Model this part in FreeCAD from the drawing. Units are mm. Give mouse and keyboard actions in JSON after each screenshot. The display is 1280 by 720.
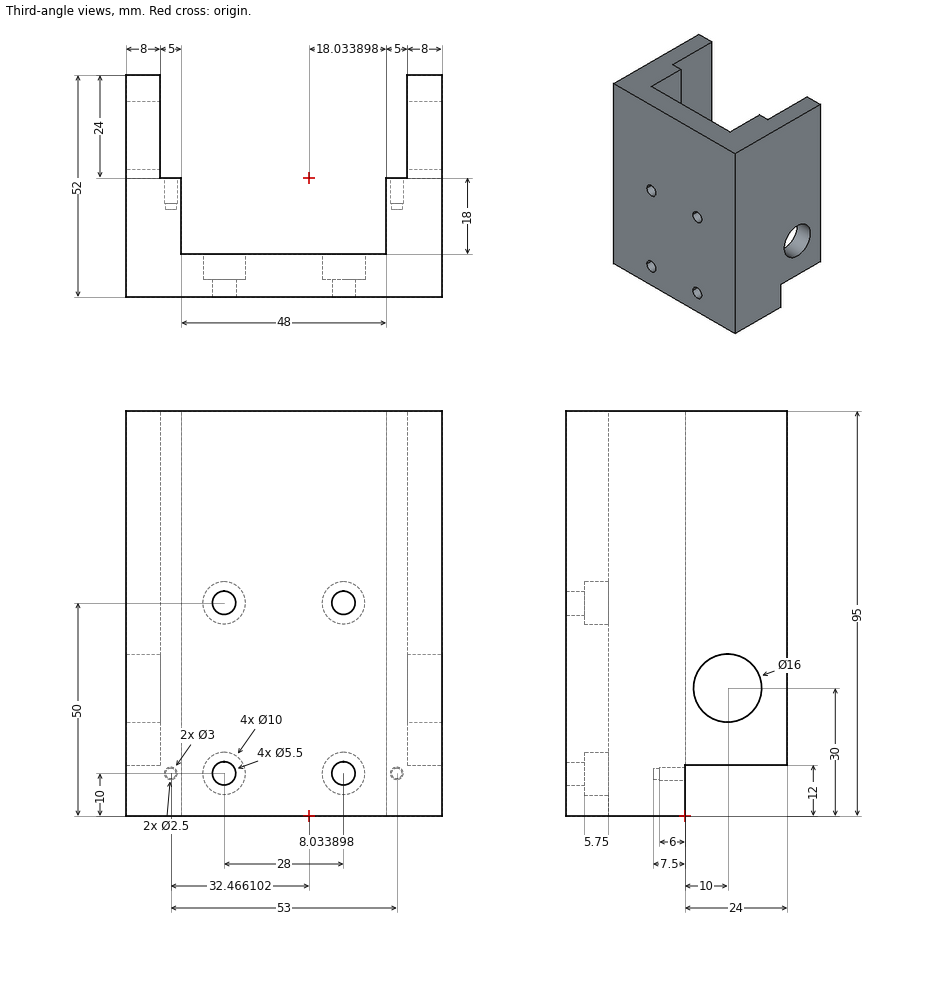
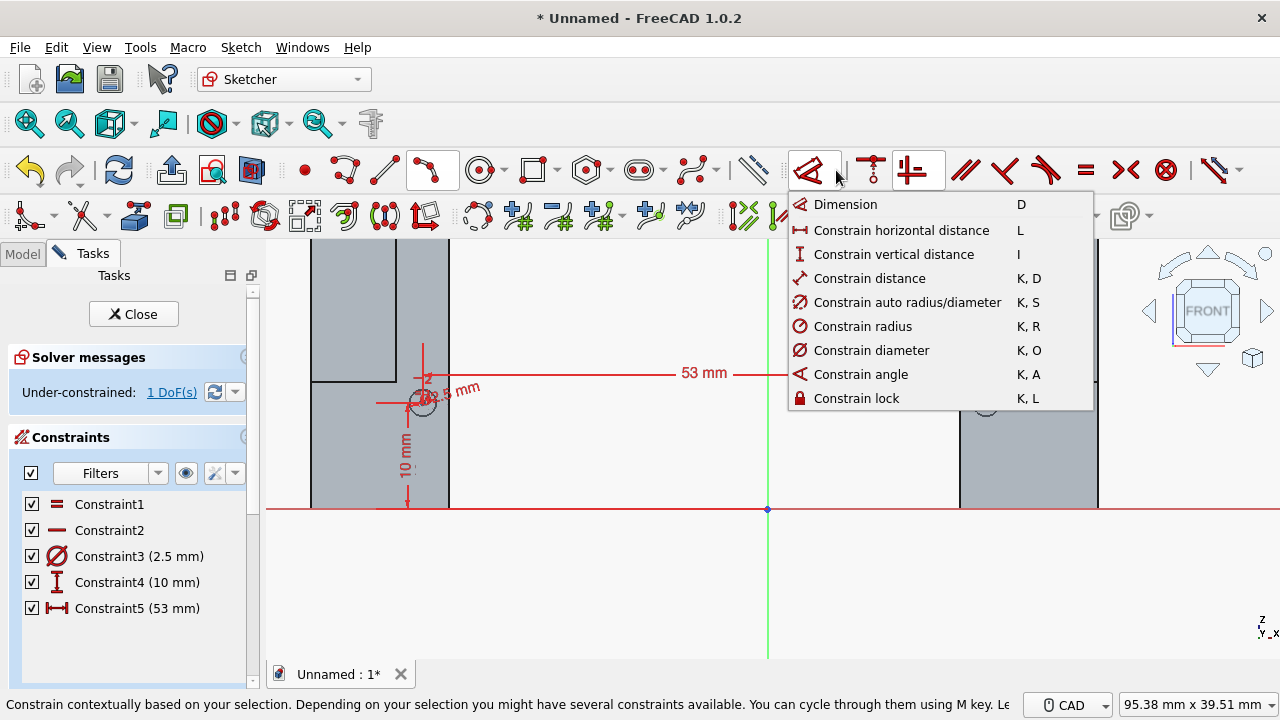
{"action": "left_click", "coordinate": [941, 230]}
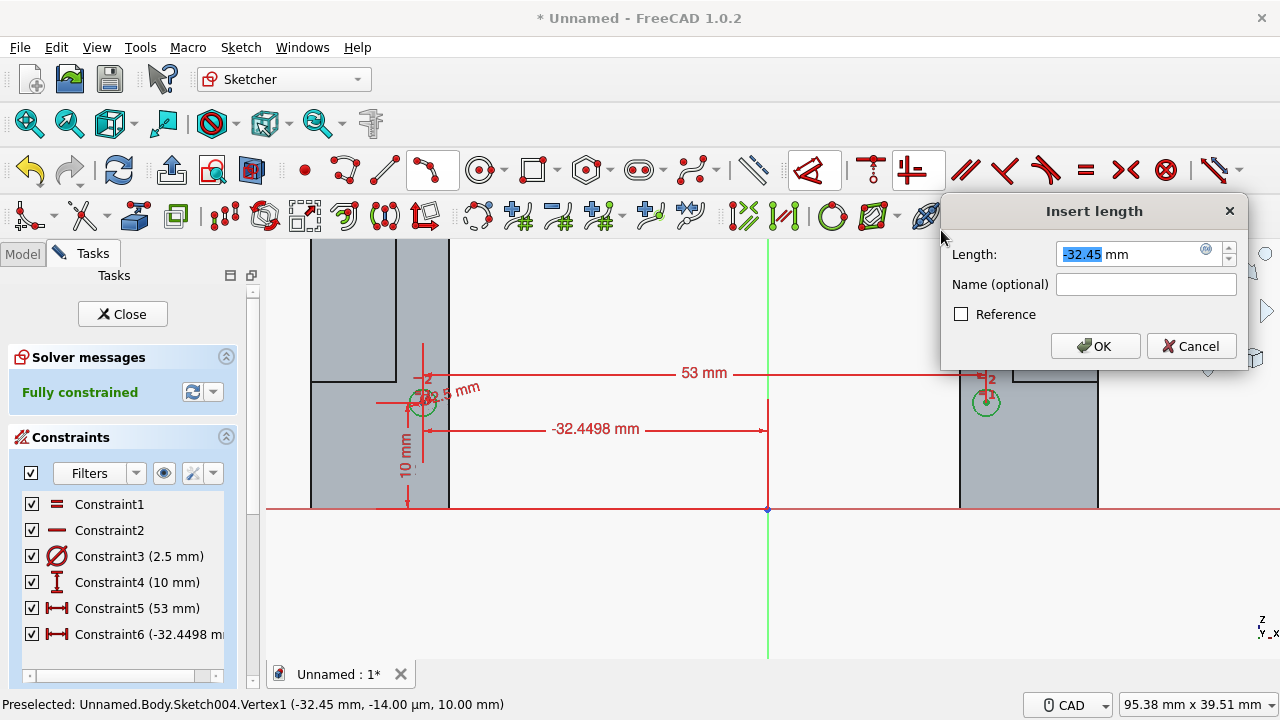
{"action": "type", "text": "-32.466102"}
{"action": "key", "text": "Return"}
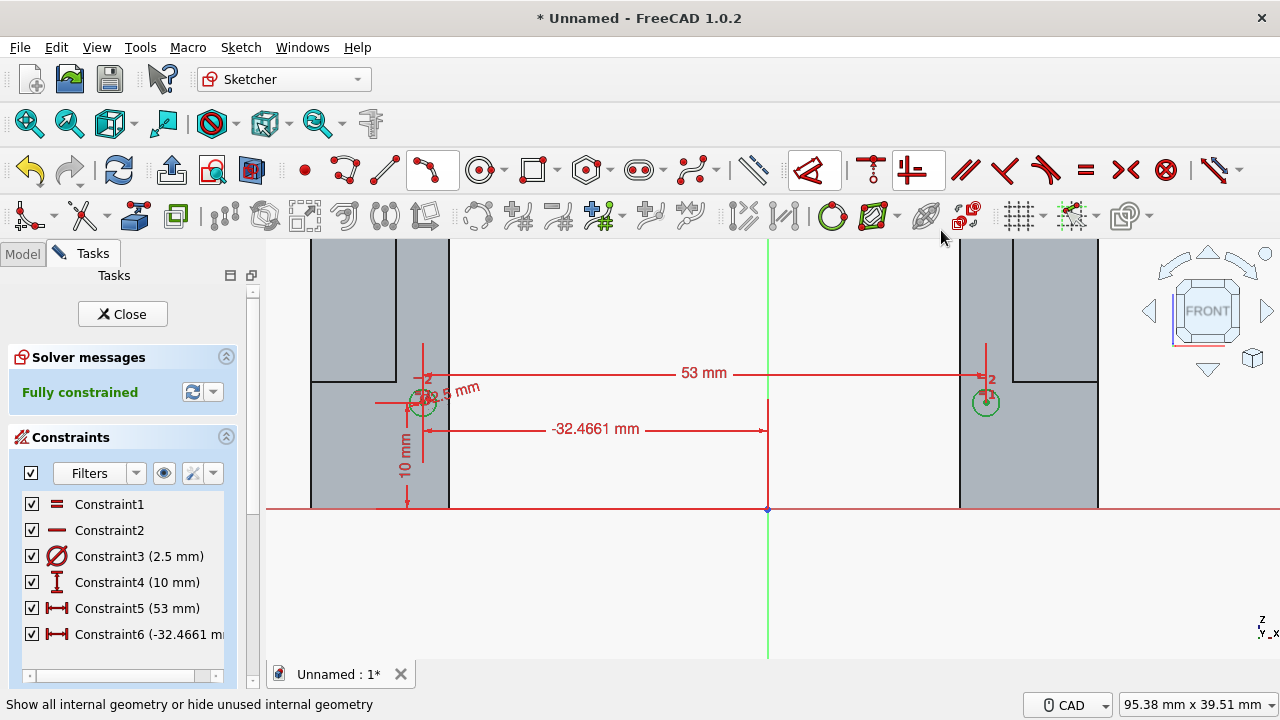
{"action": "left_click", "coordinate": [123, 314]}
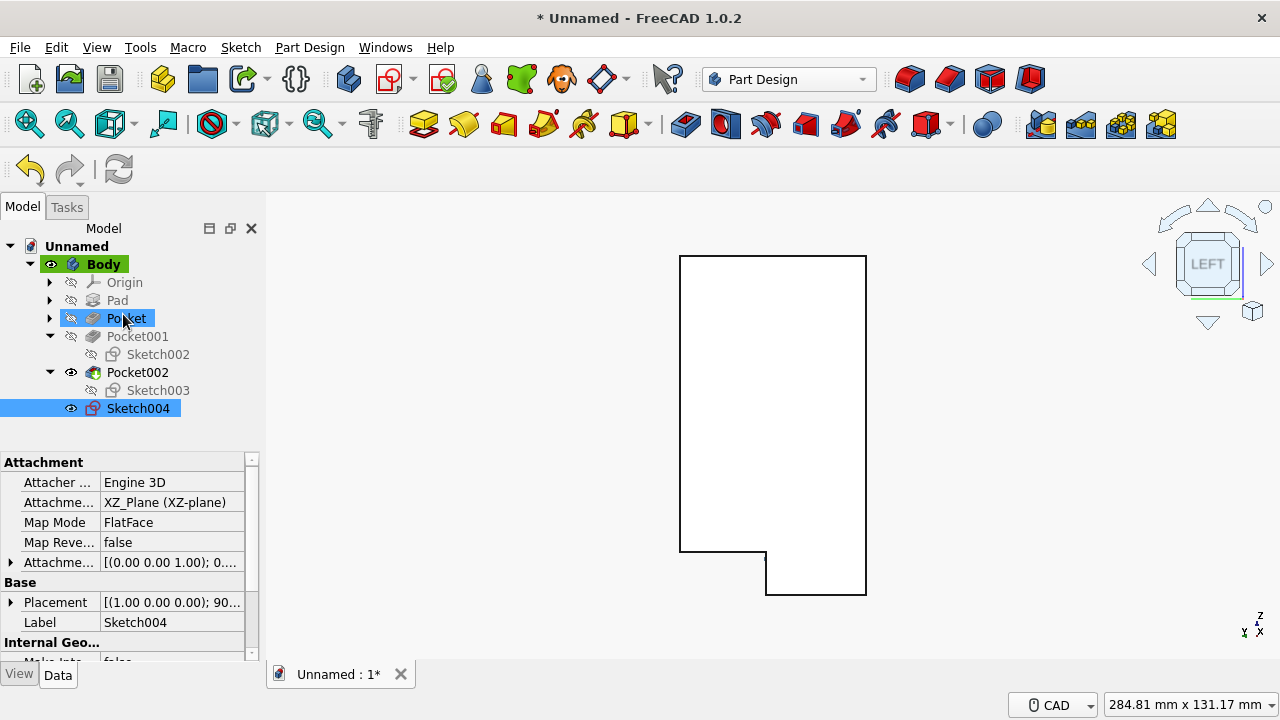
{"action": "left_click", "coordinate": [686, 124]}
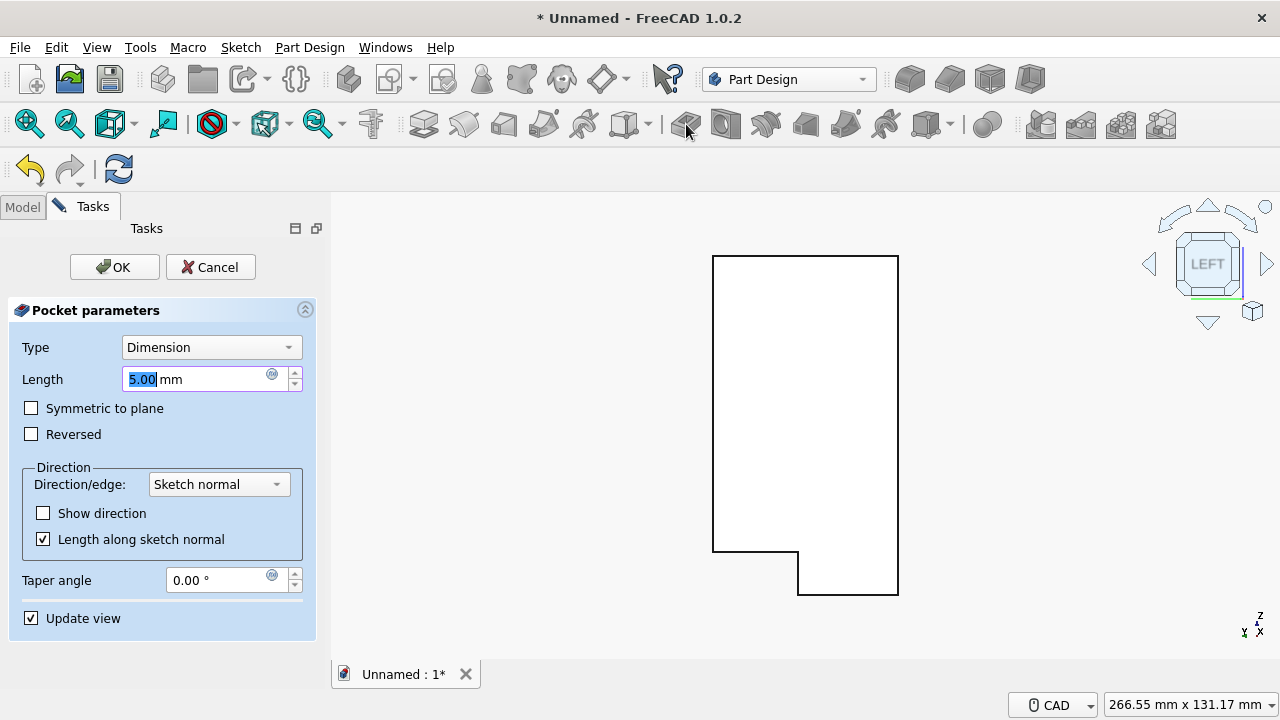
{"action": "type", "text": "7.5"}
{"action": "key", "text": "Tab"}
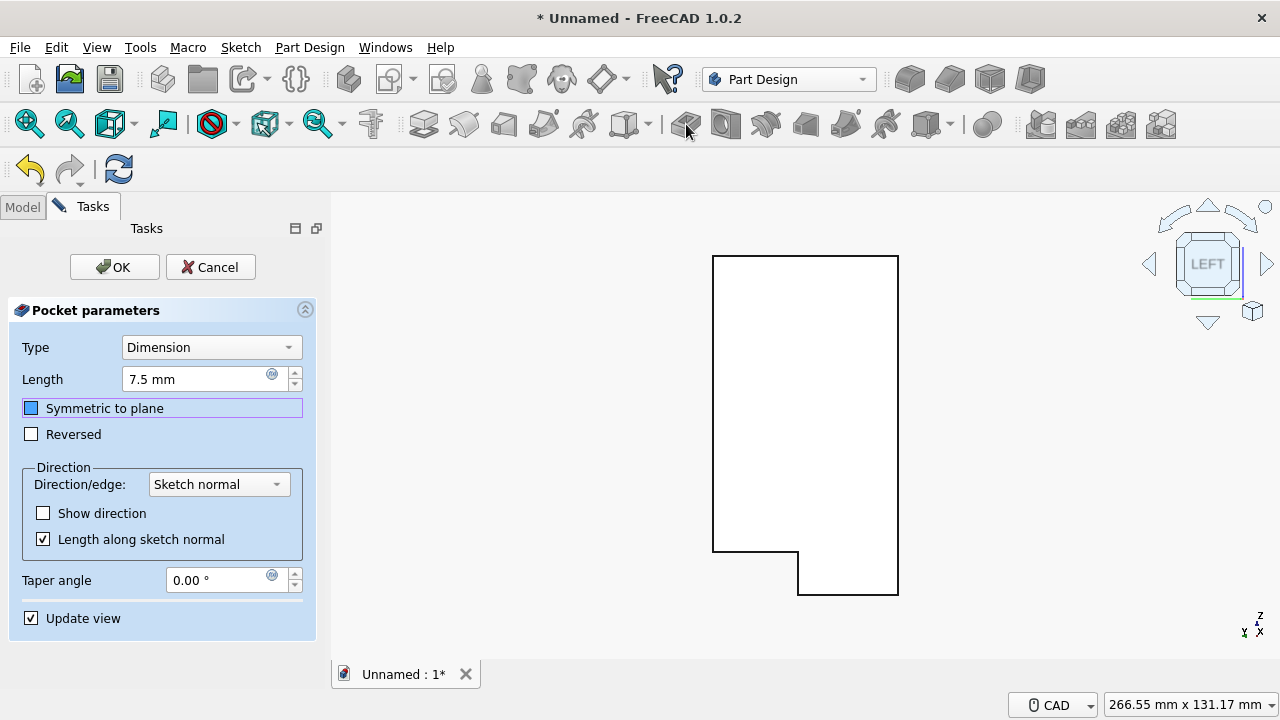
{"action": "left_click", "coordinate": [30, 434]}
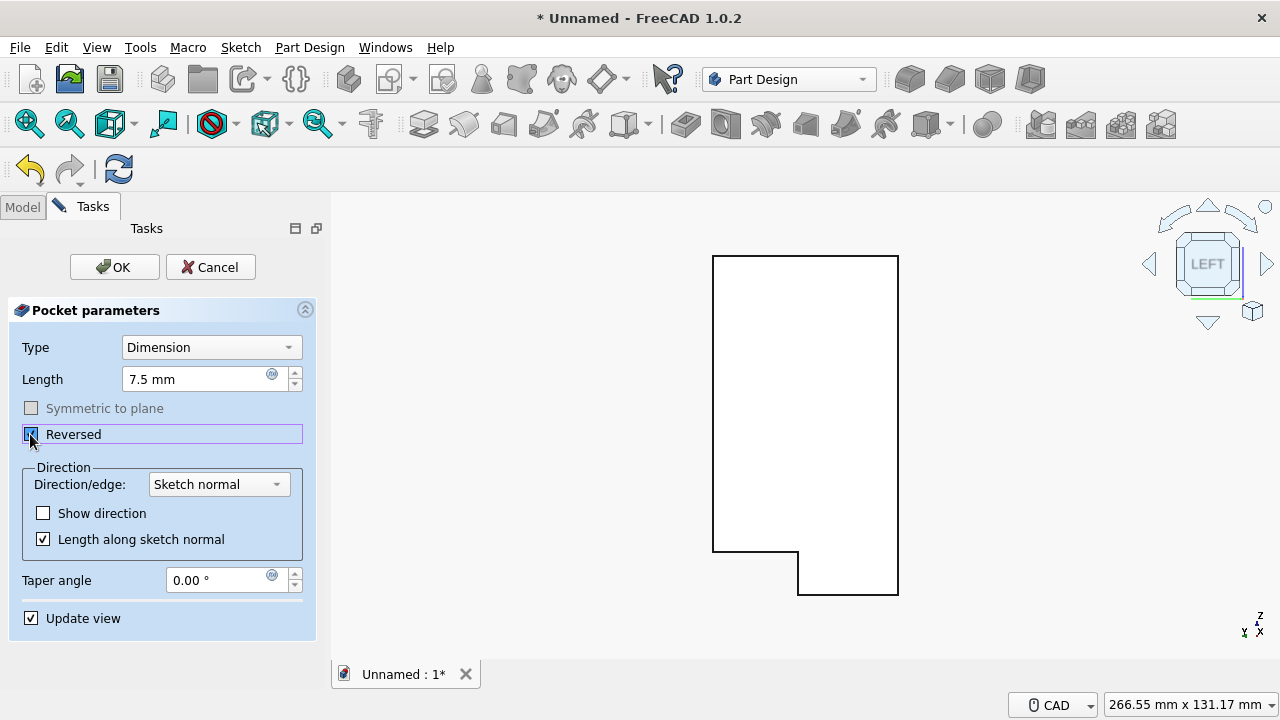
{"action": "left_click", "coordinate": [115, 267]}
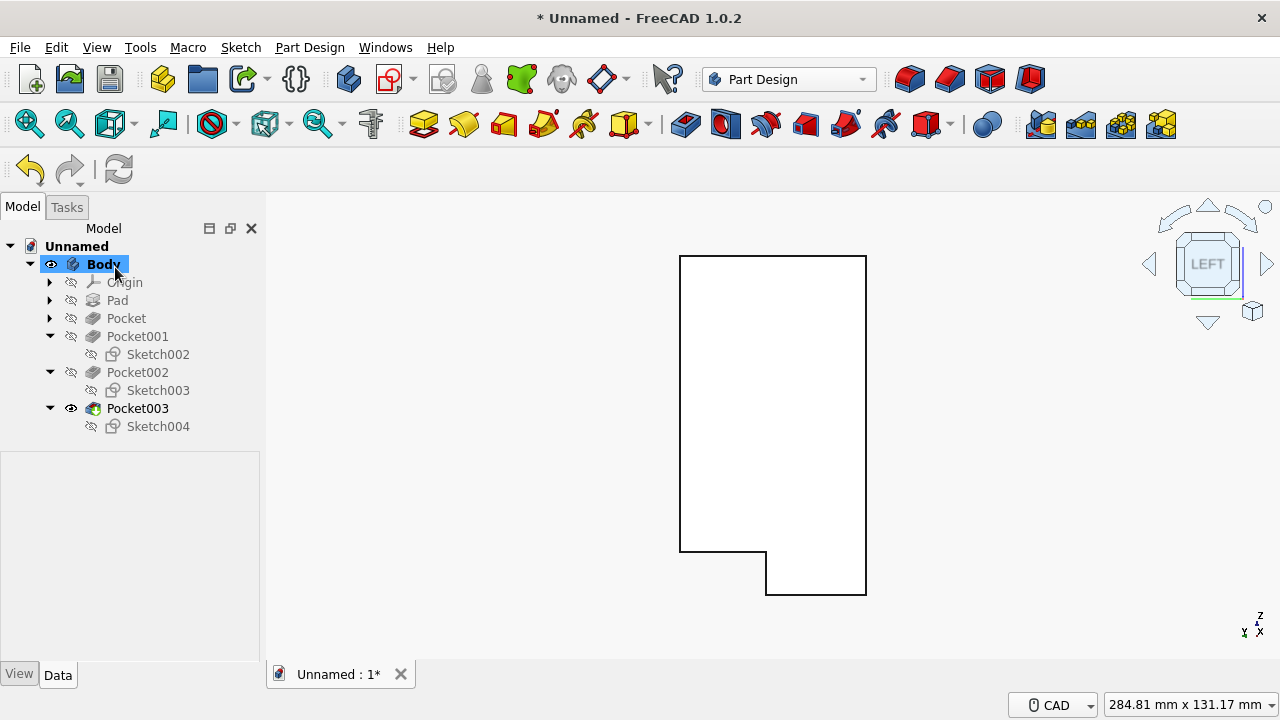
{"action": "key", "text": "4"}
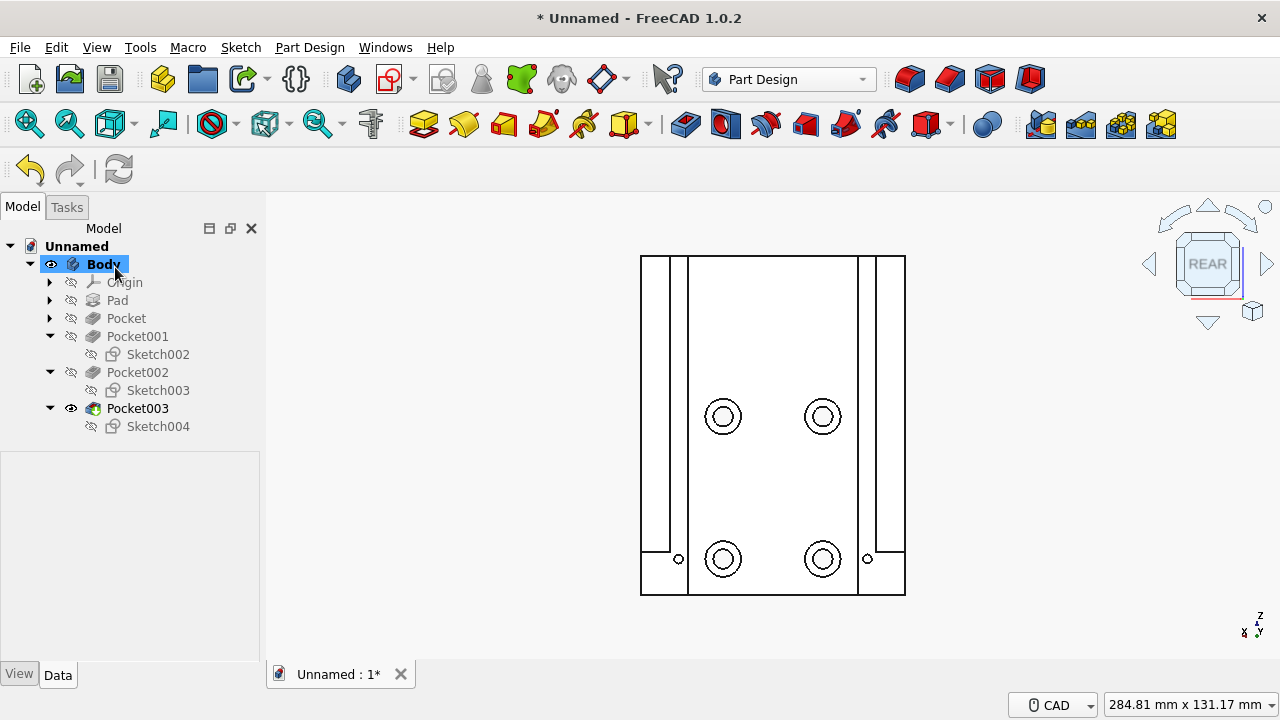
{"action": "left_click", "coordinate": [658, 569]}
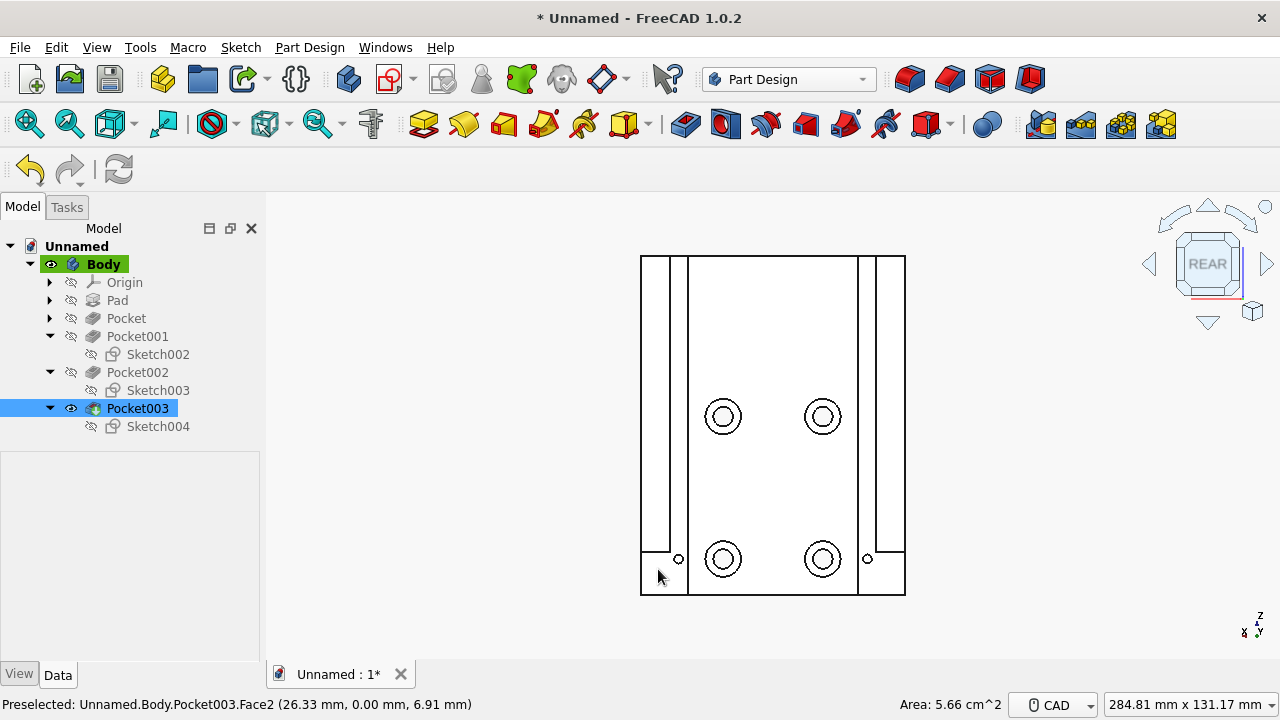
{"action": "left_click", "coordinate": [390, 80]}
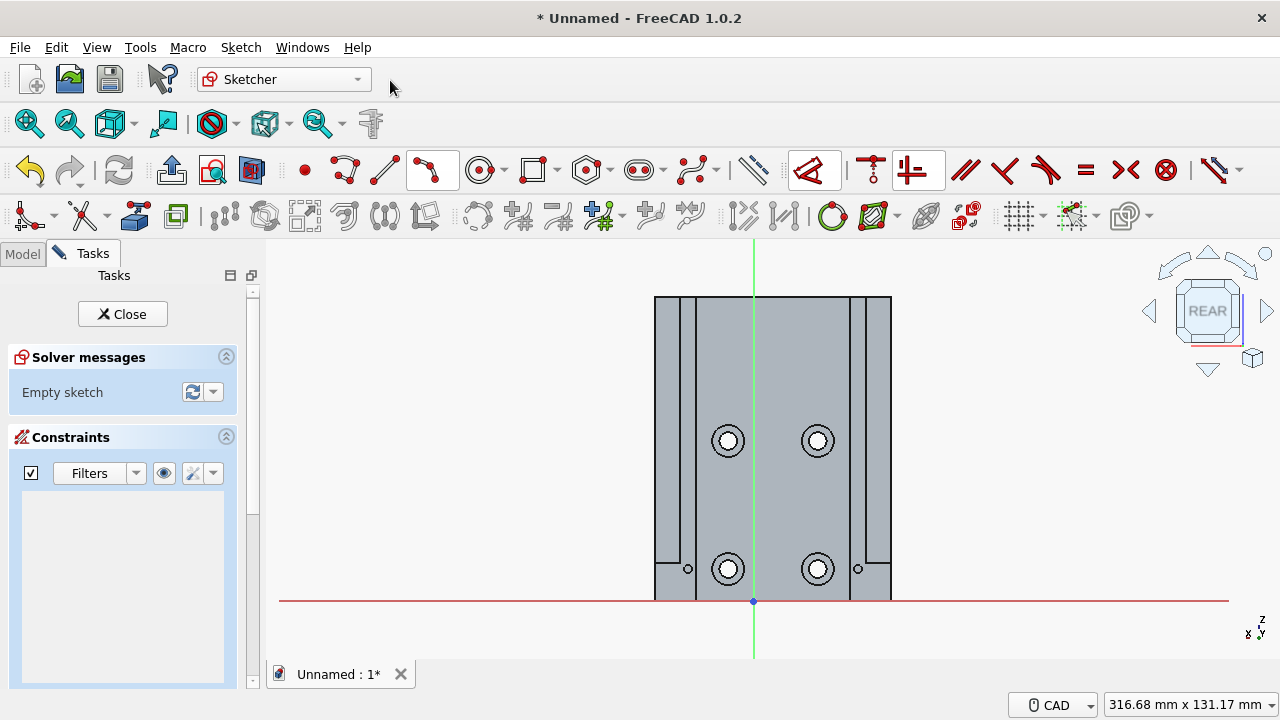
{"action": "key", "text": "q s"}